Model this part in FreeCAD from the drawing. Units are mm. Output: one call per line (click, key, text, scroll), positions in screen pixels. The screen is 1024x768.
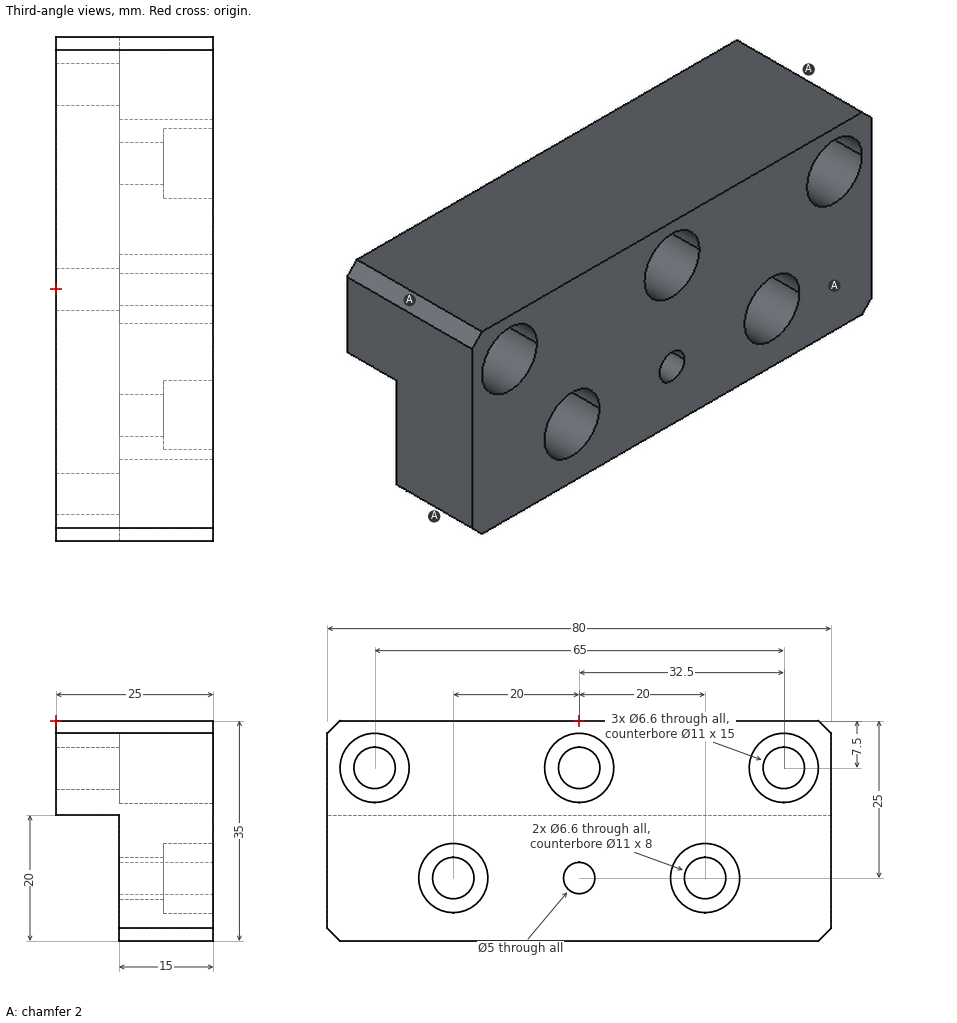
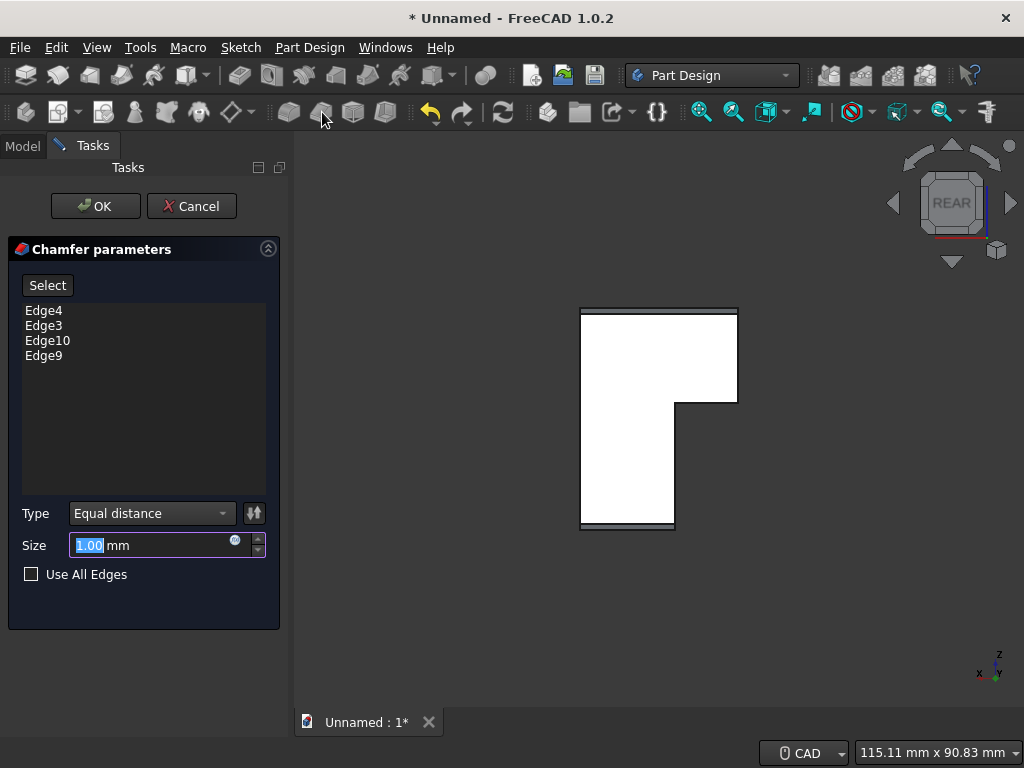
text(2)
key(Tab)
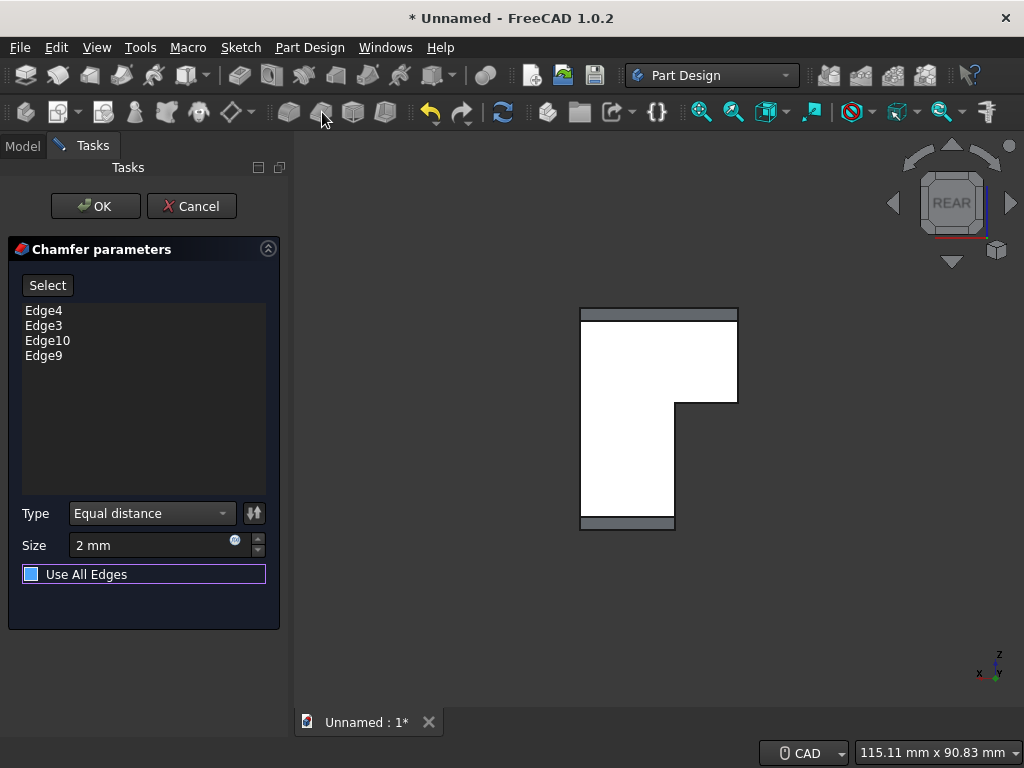
click(96, 206)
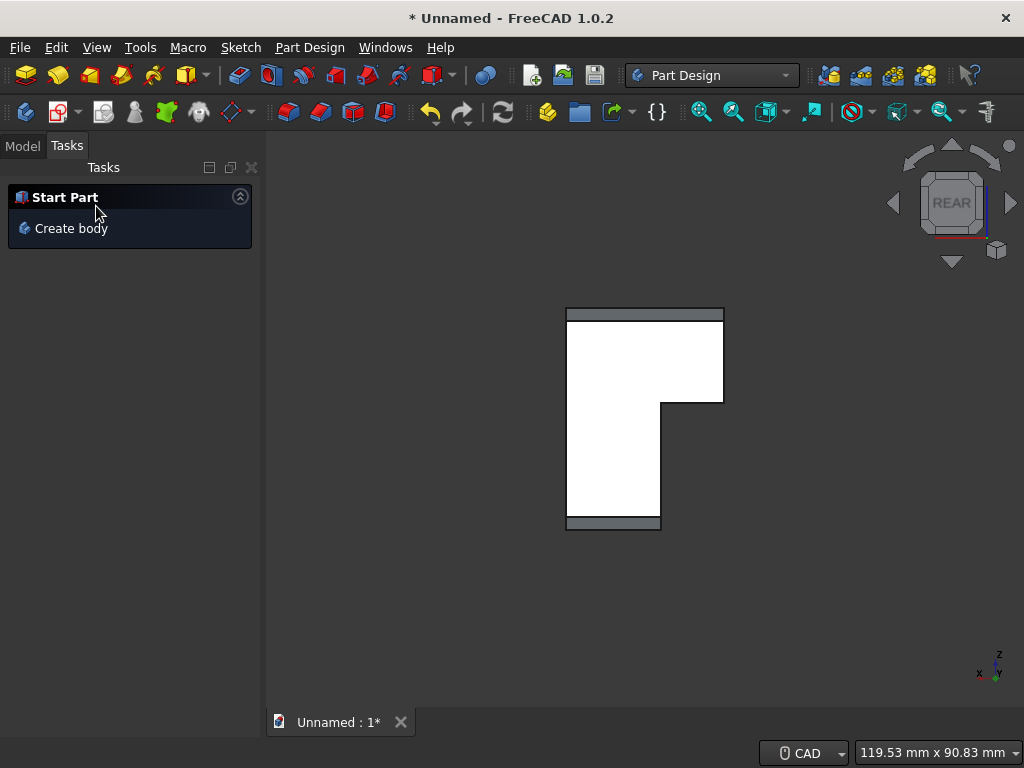
click(702, 112)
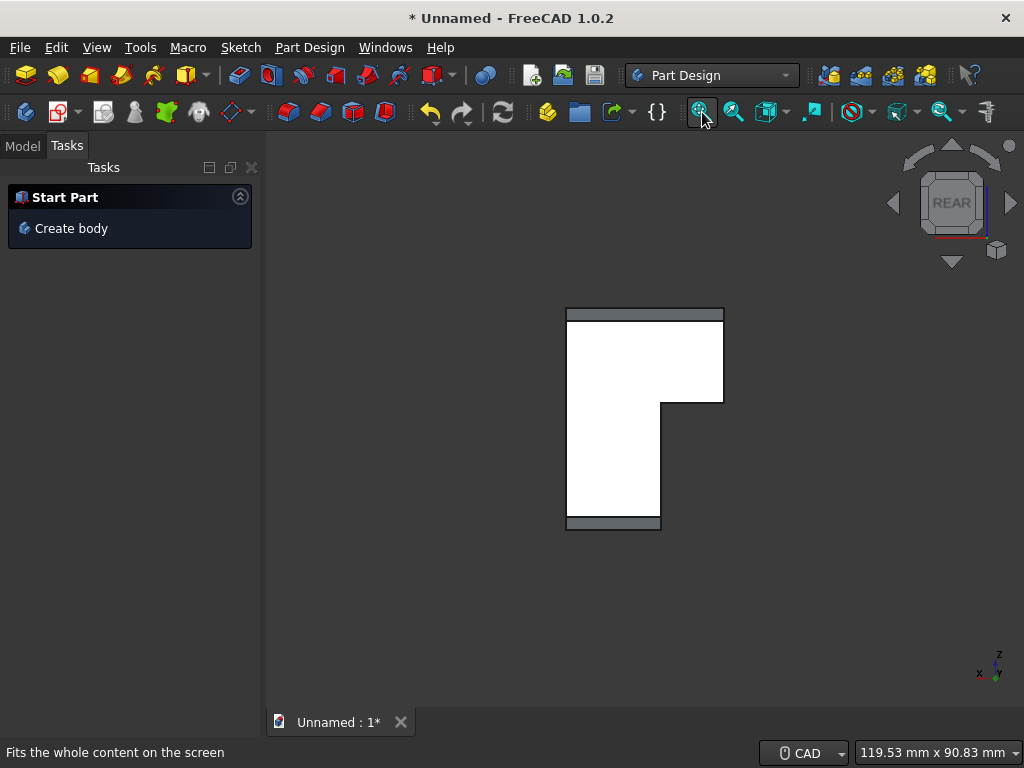
key(0)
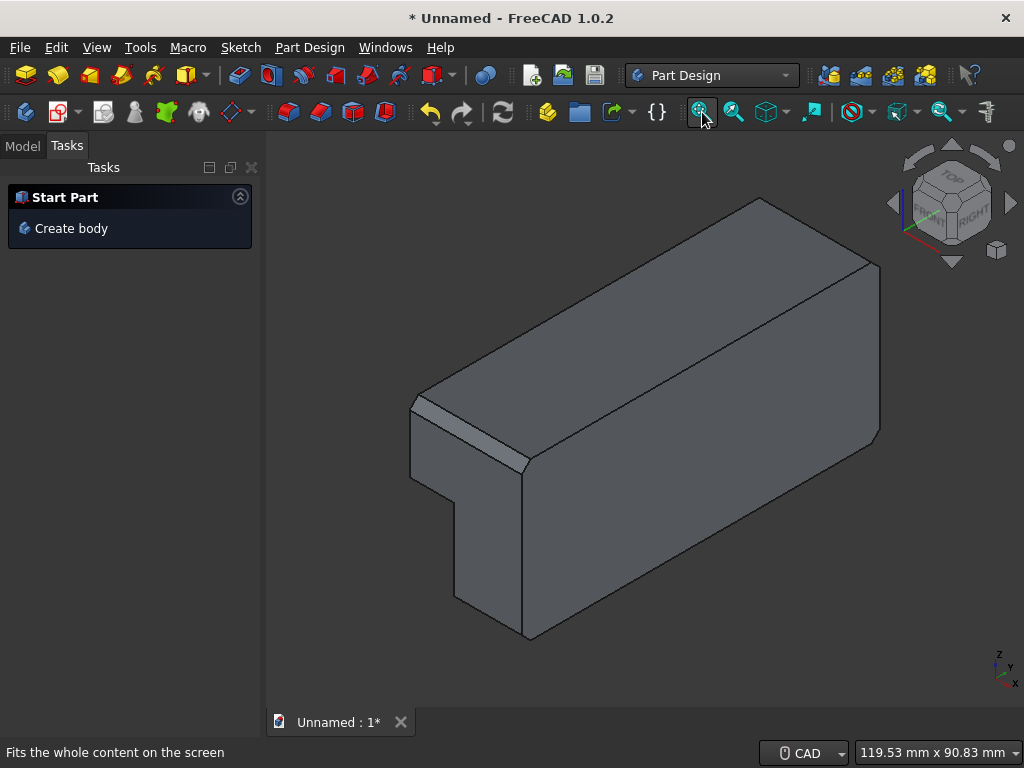
click(701, 450)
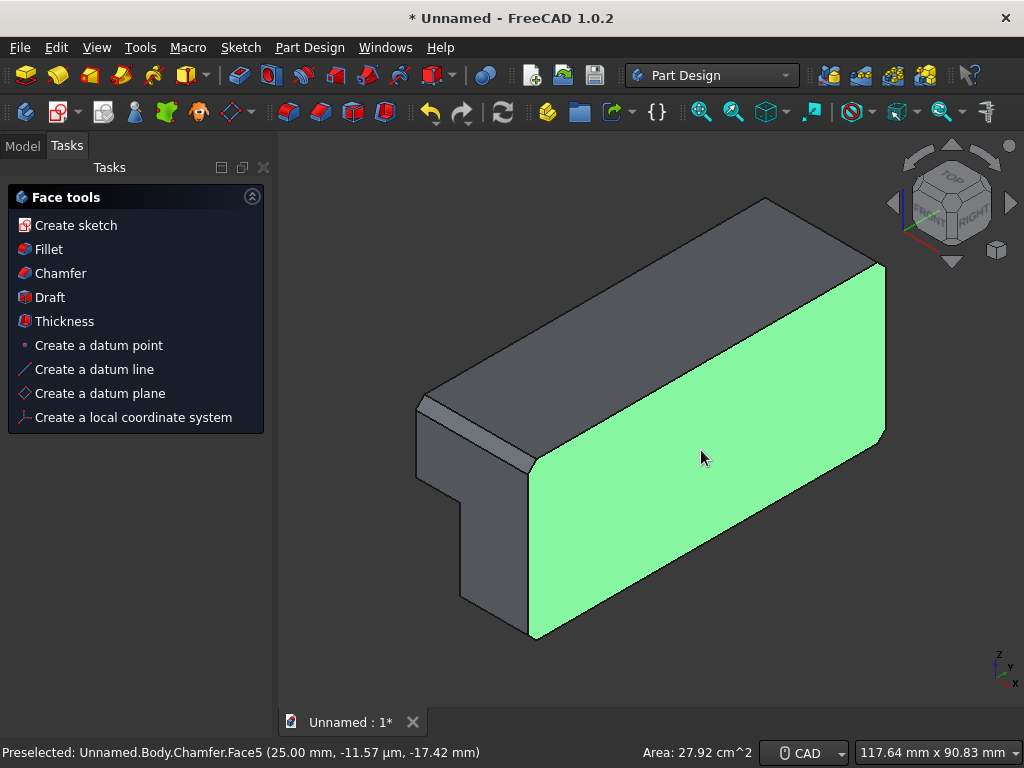
click(58, 112)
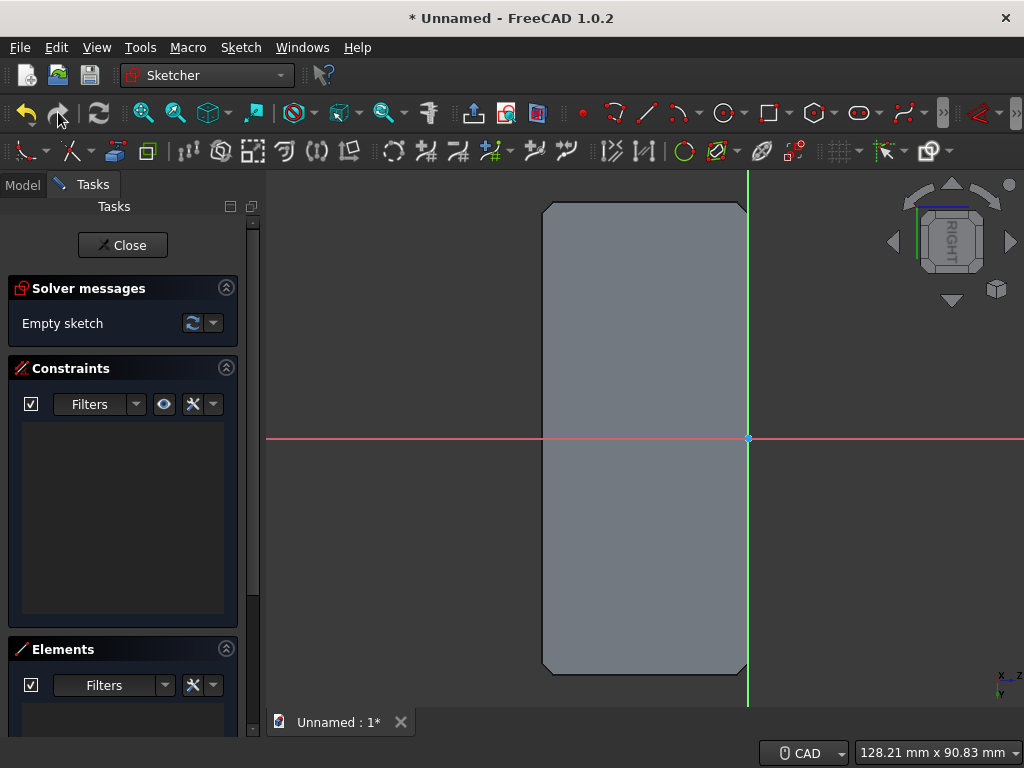
click(724, 114)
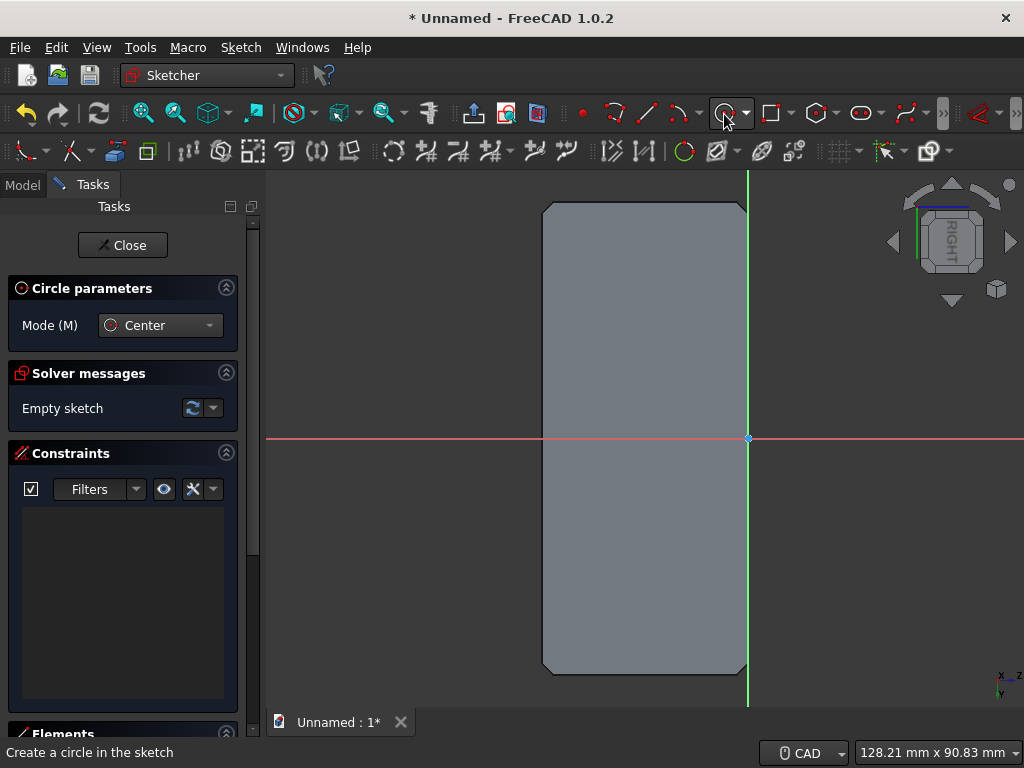
click(704, 631)
click(718, 617)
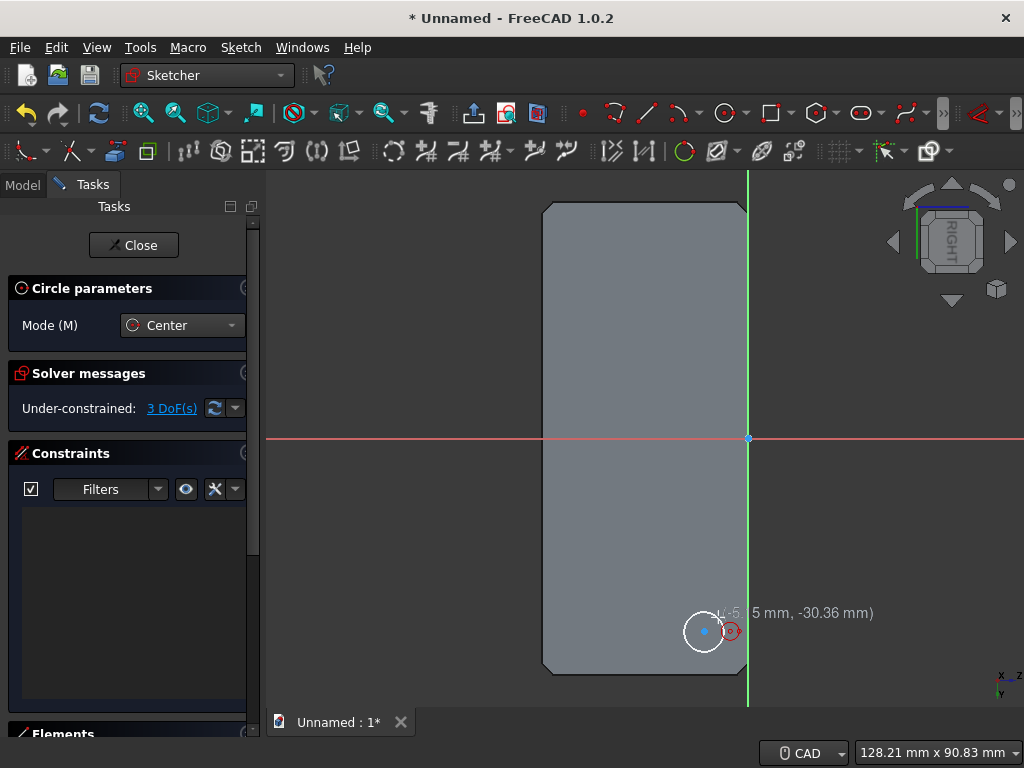
click(704, 438)
click(711, 420)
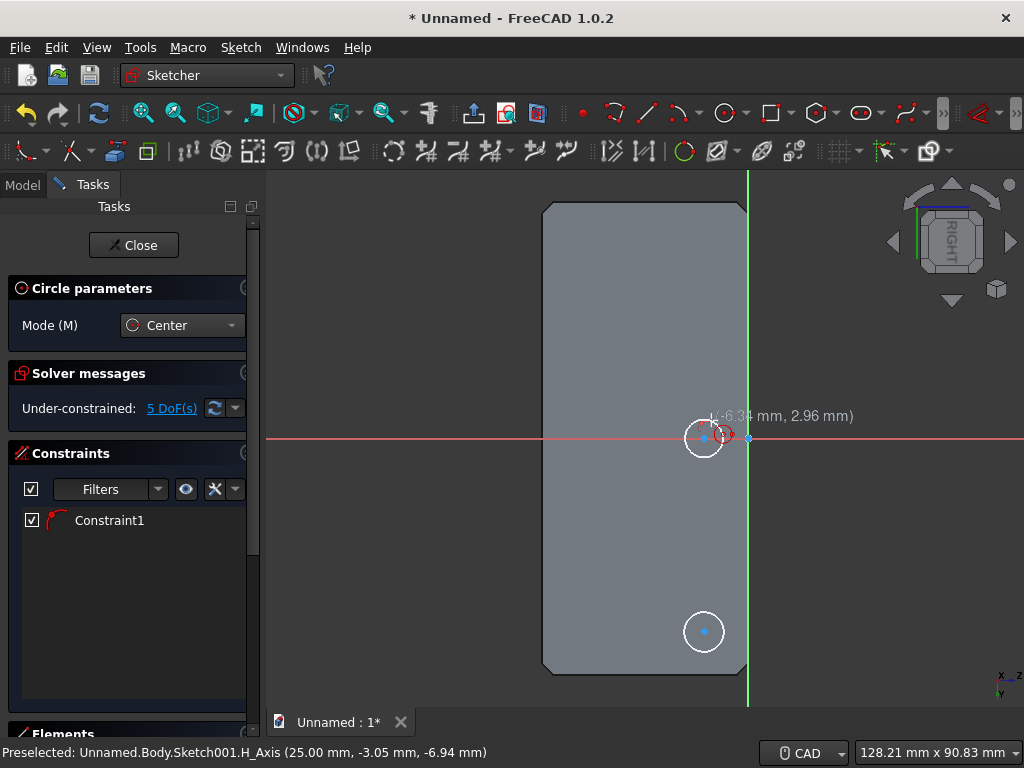
click(704, 246)
click(718, 233)
key(Escape)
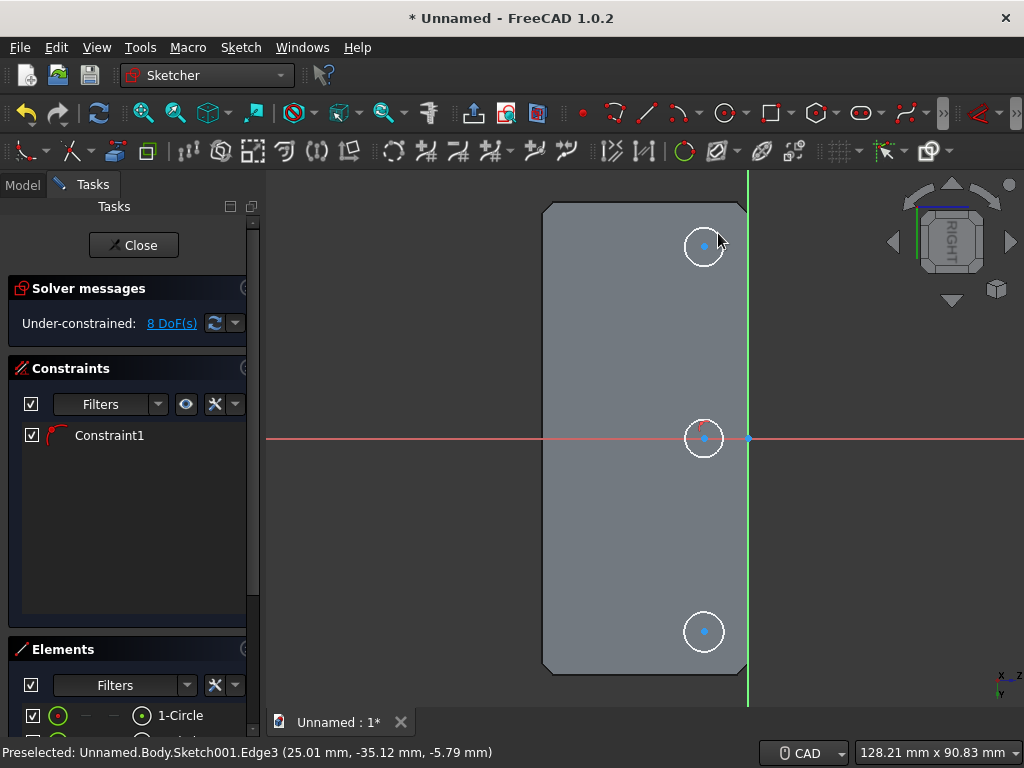
click(718, 618)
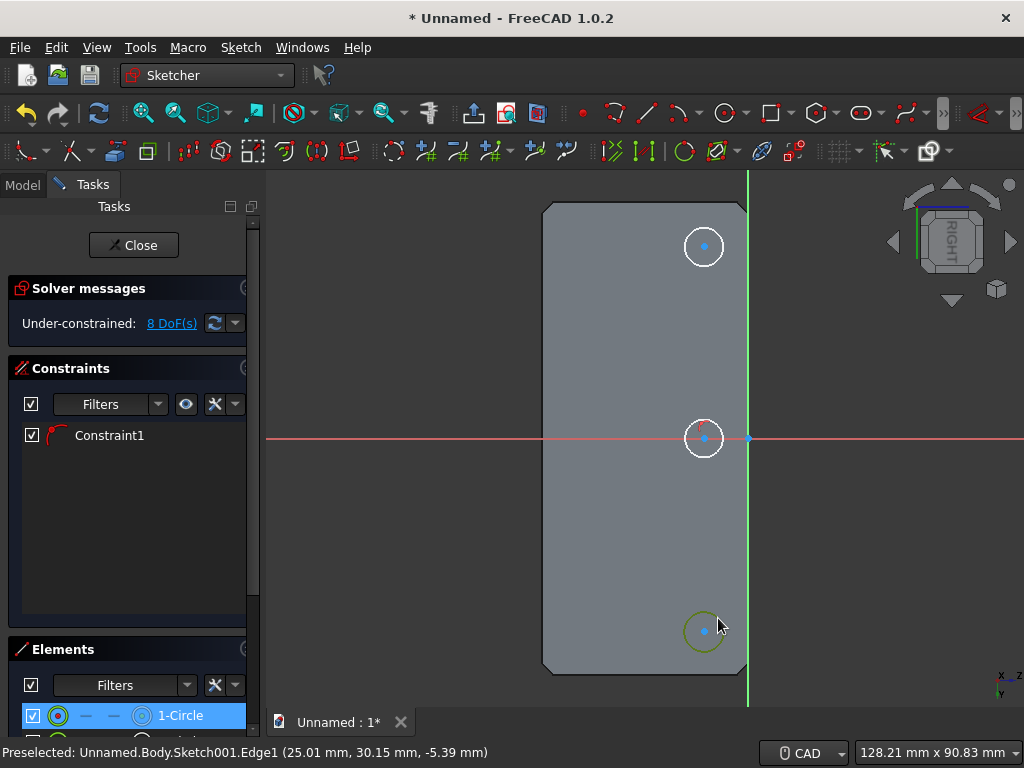
click(717, 425)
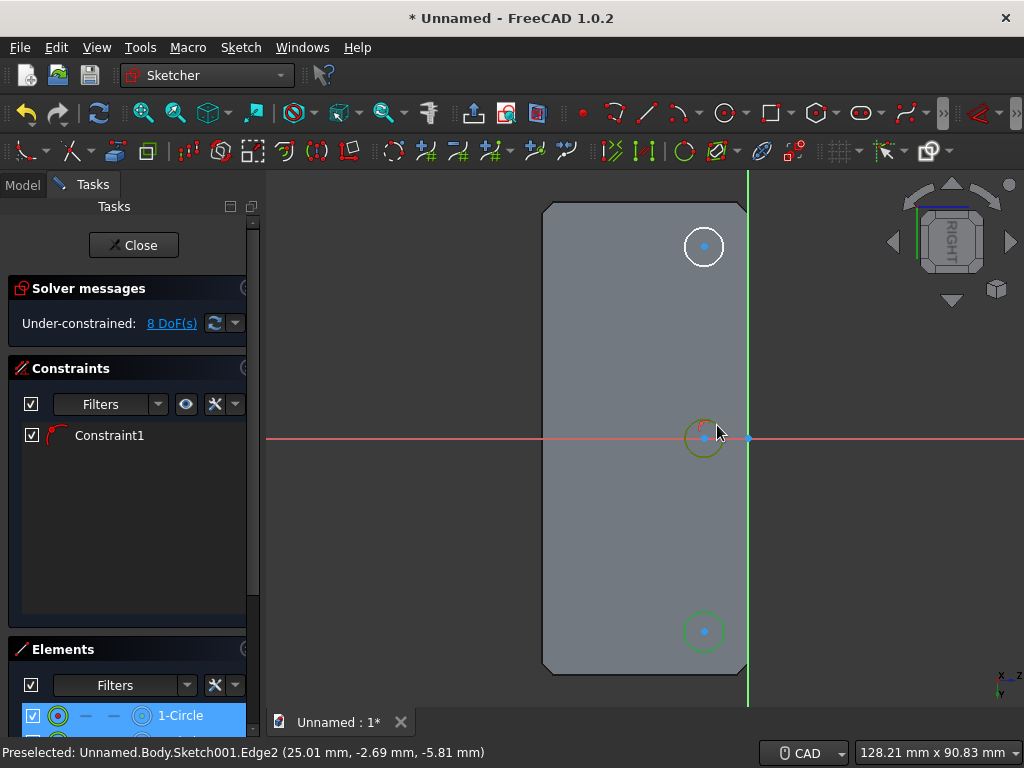
click(717, 233)